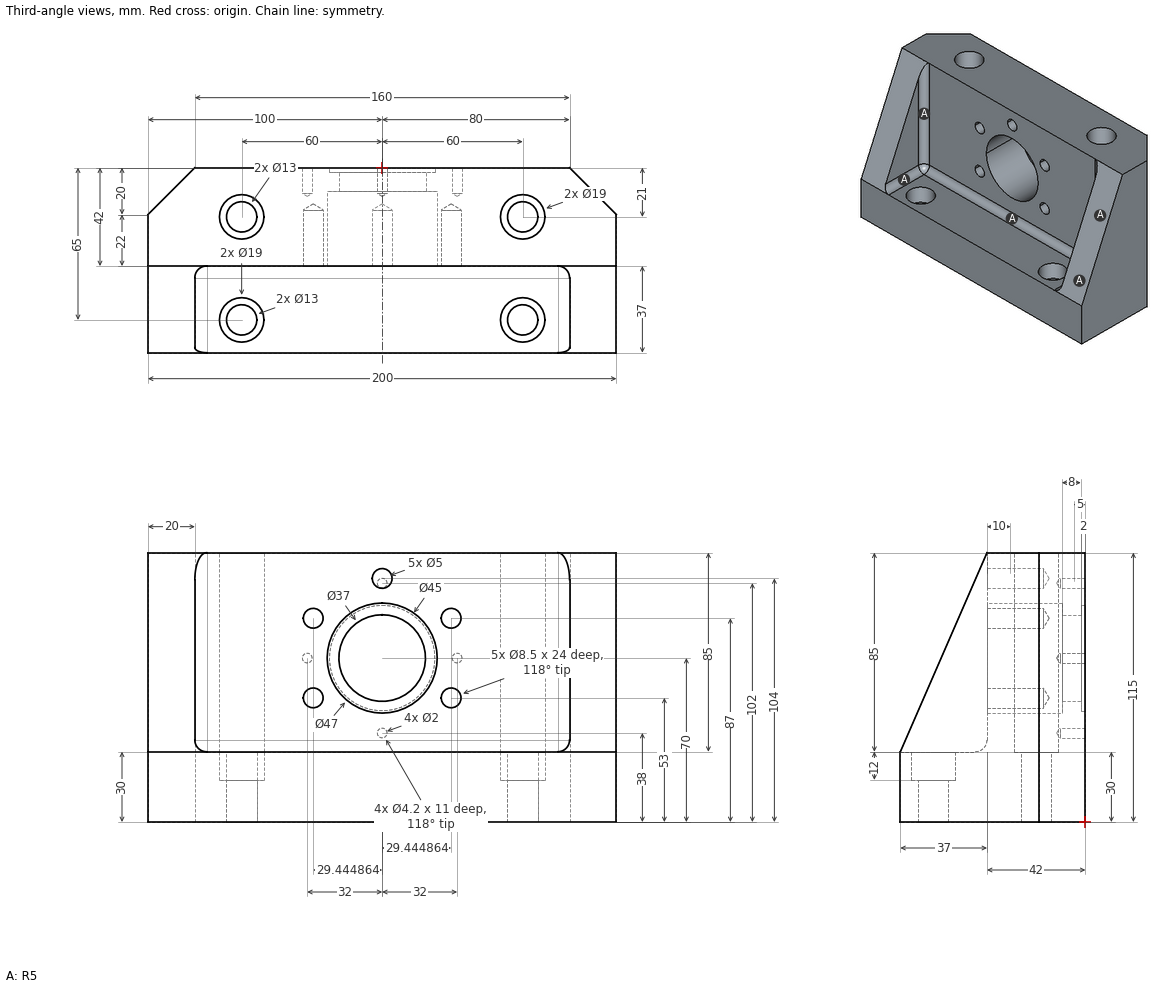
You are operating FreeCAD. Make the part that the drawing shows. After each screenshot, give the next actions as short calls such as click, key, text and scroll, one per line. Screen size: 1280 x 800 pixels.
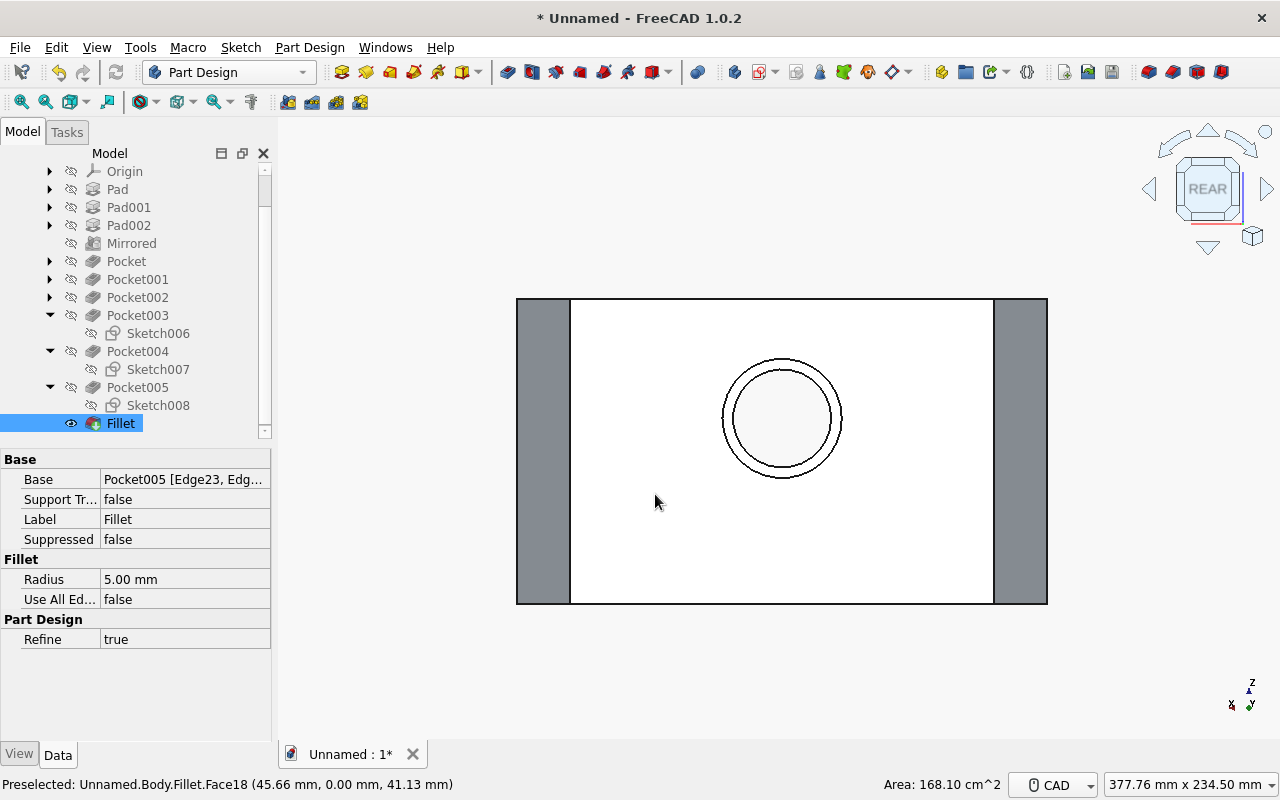
click(760, 72)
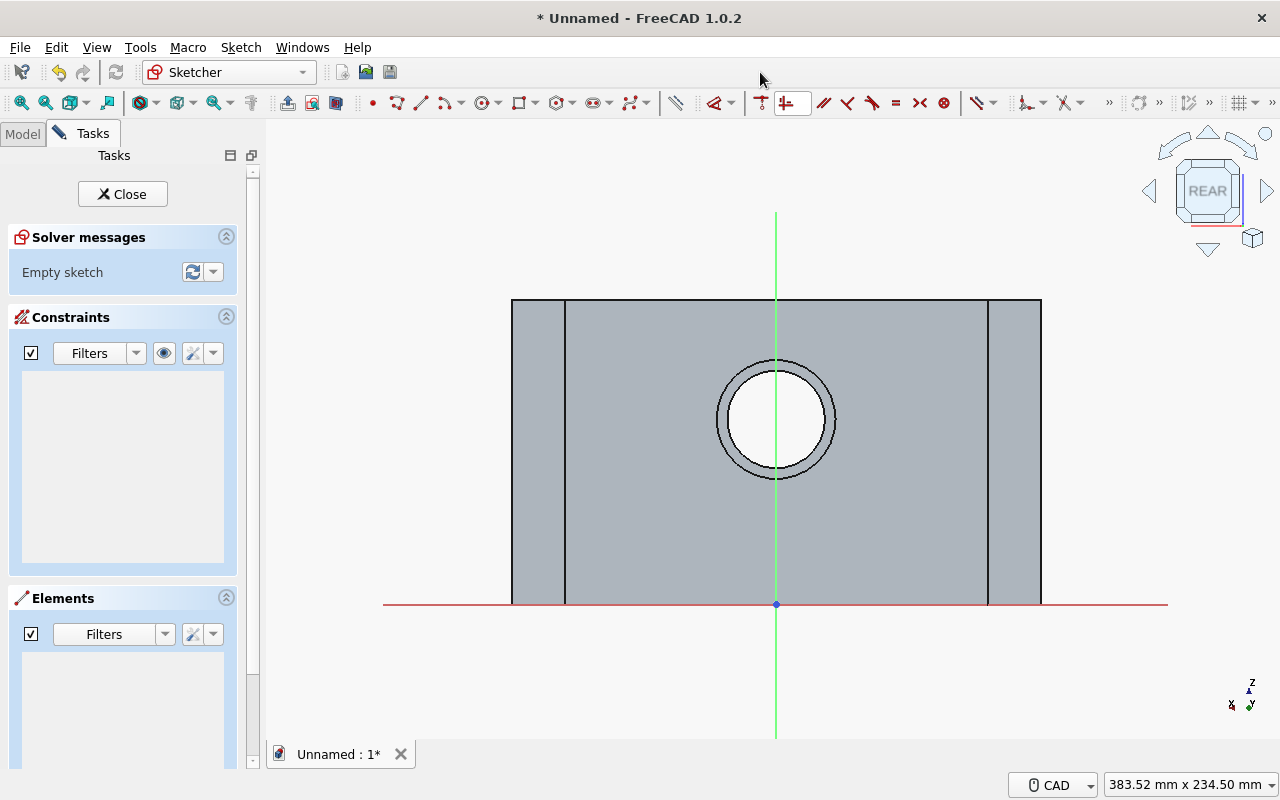
scroll(922, 548, up, 2)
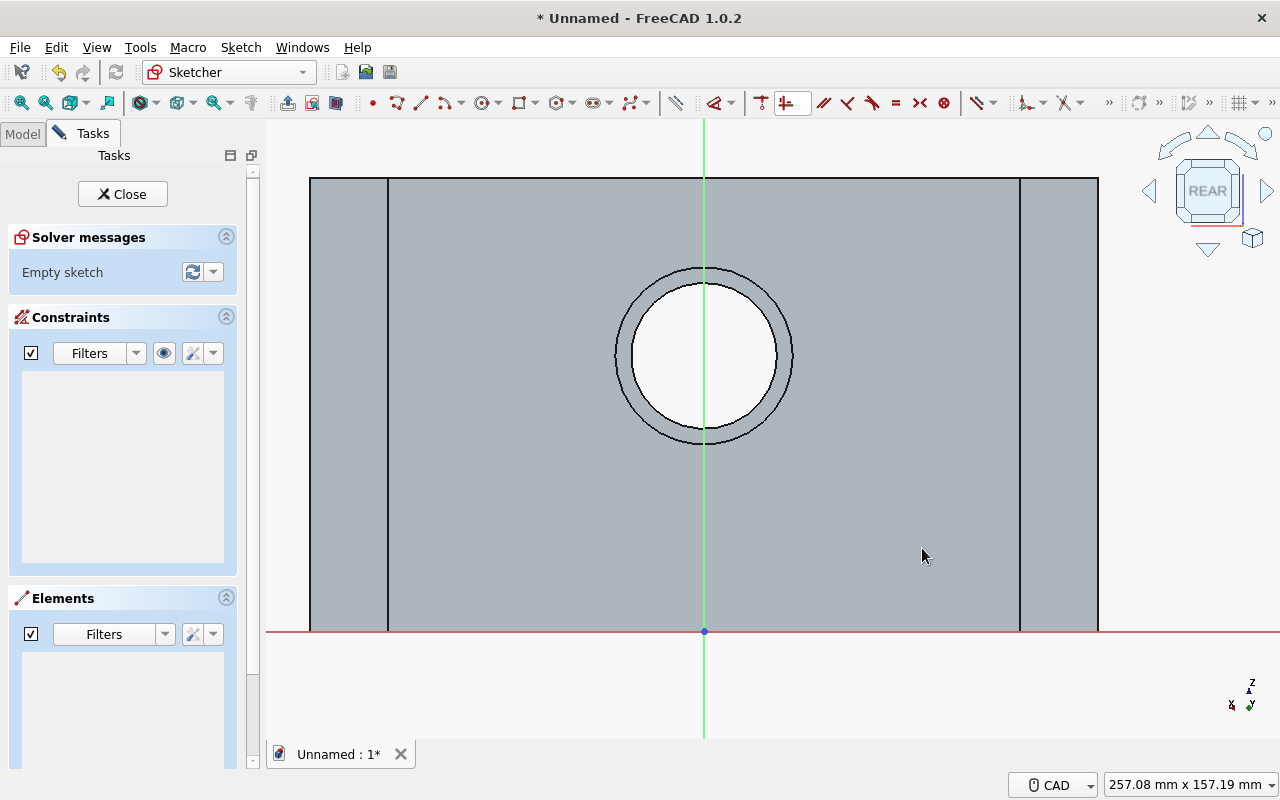
click(482, 104)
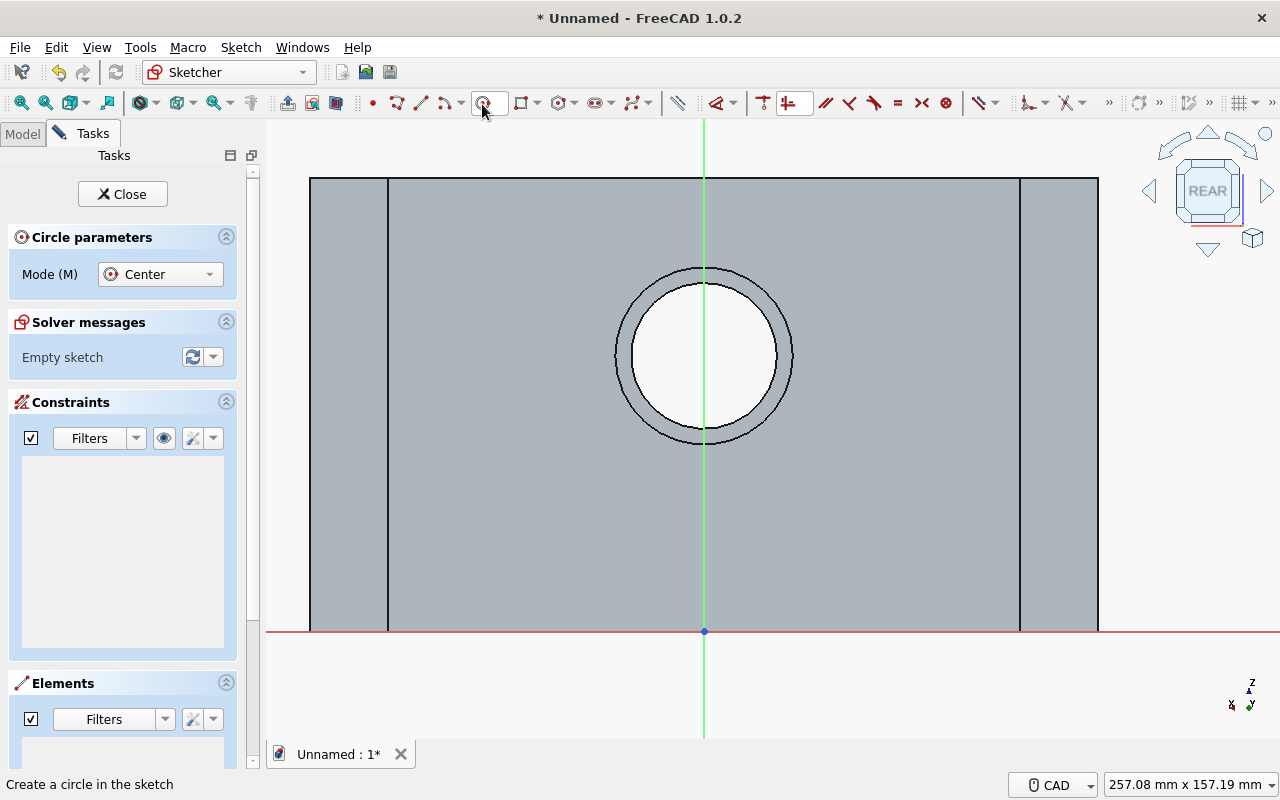
scroll(704, 482, up, 9)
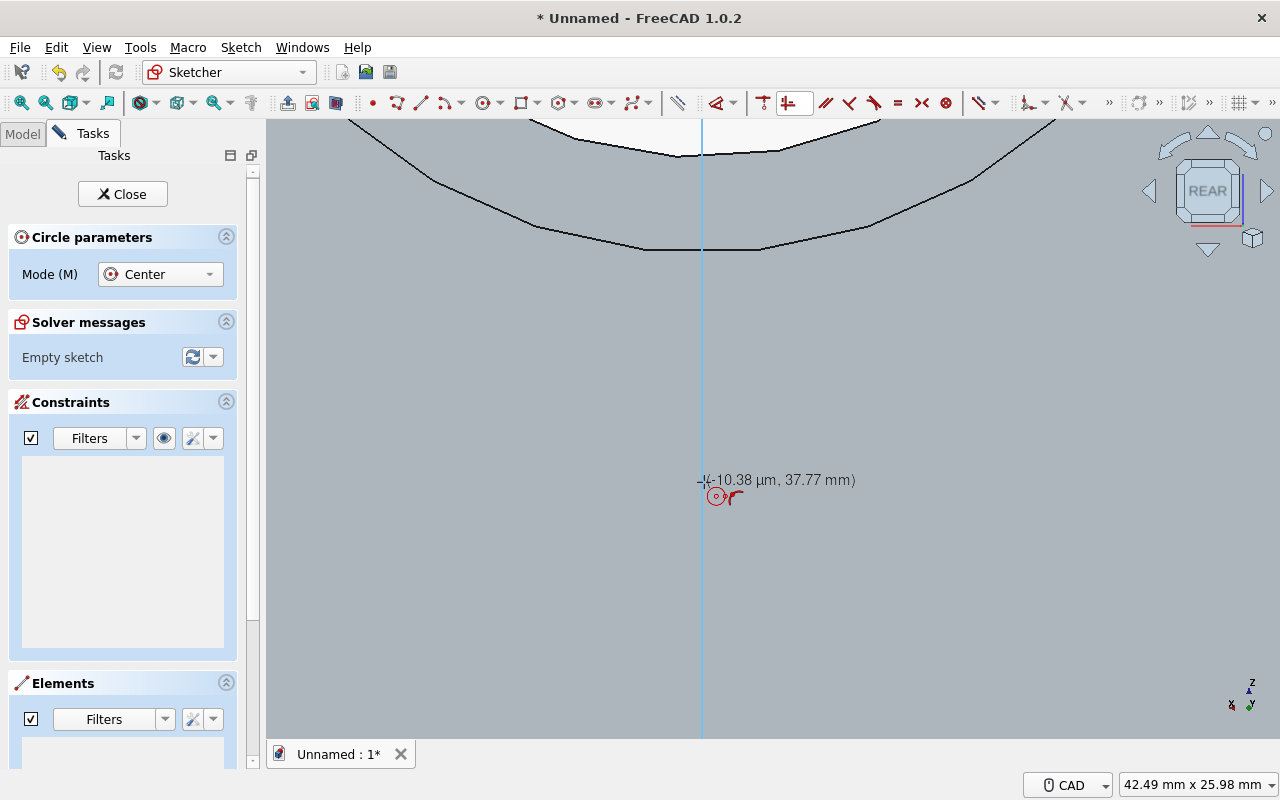
scroll(705, 483, down, 9)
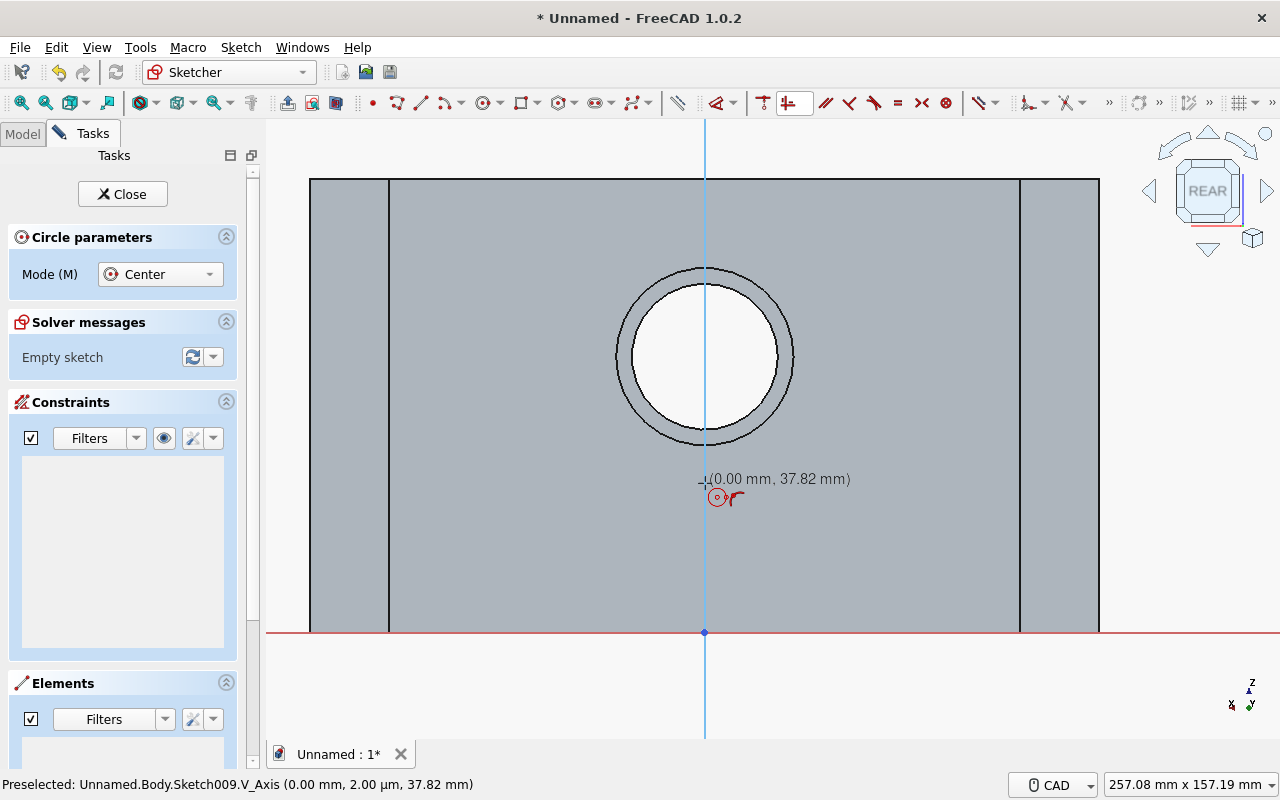
click(705, 483)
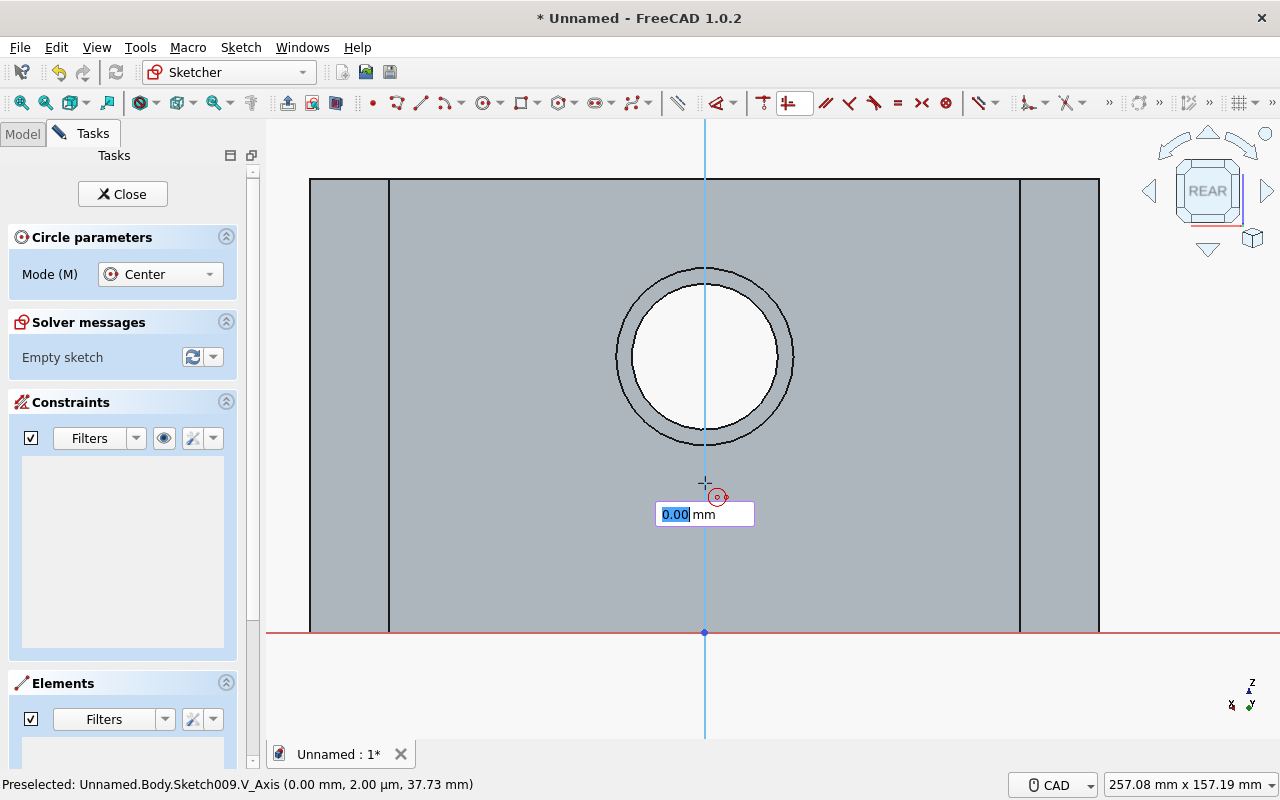
scroll(709, 482, up, 8)
move(705, 478)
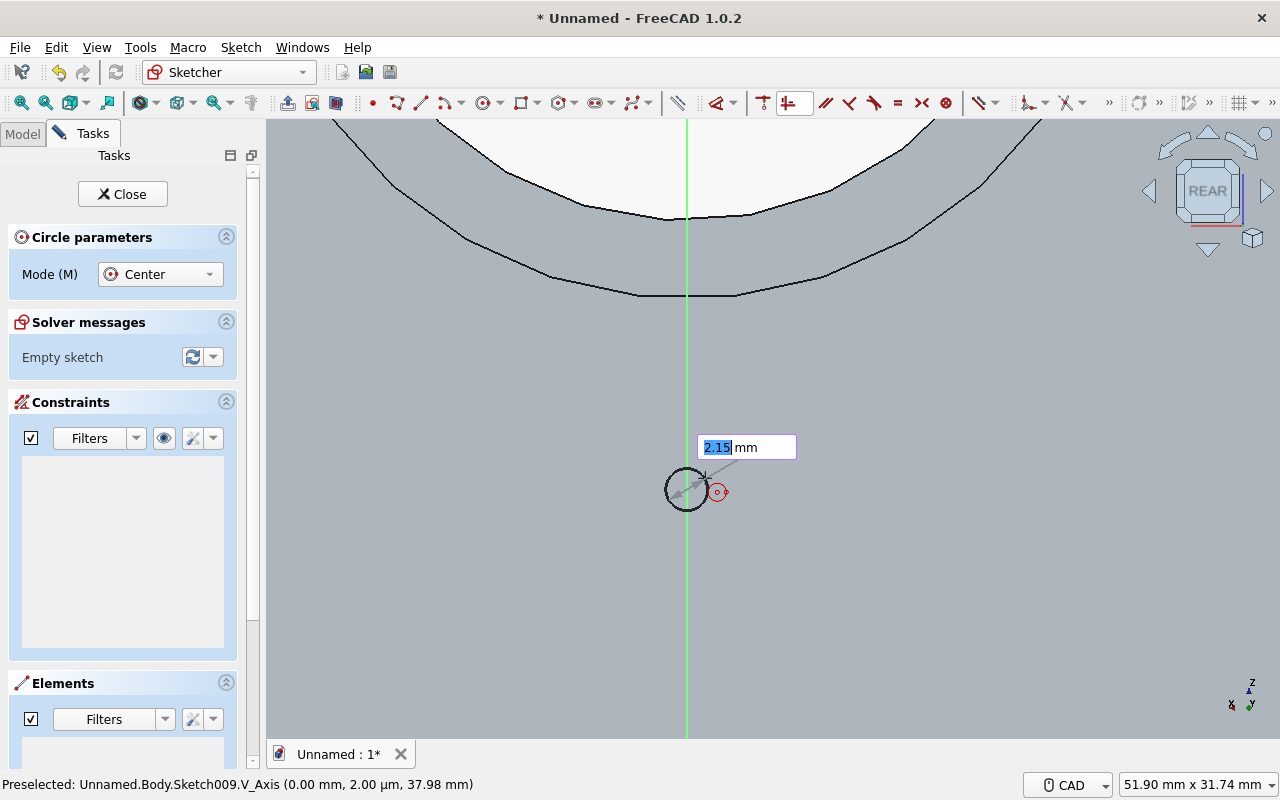
text(2)
key(Return)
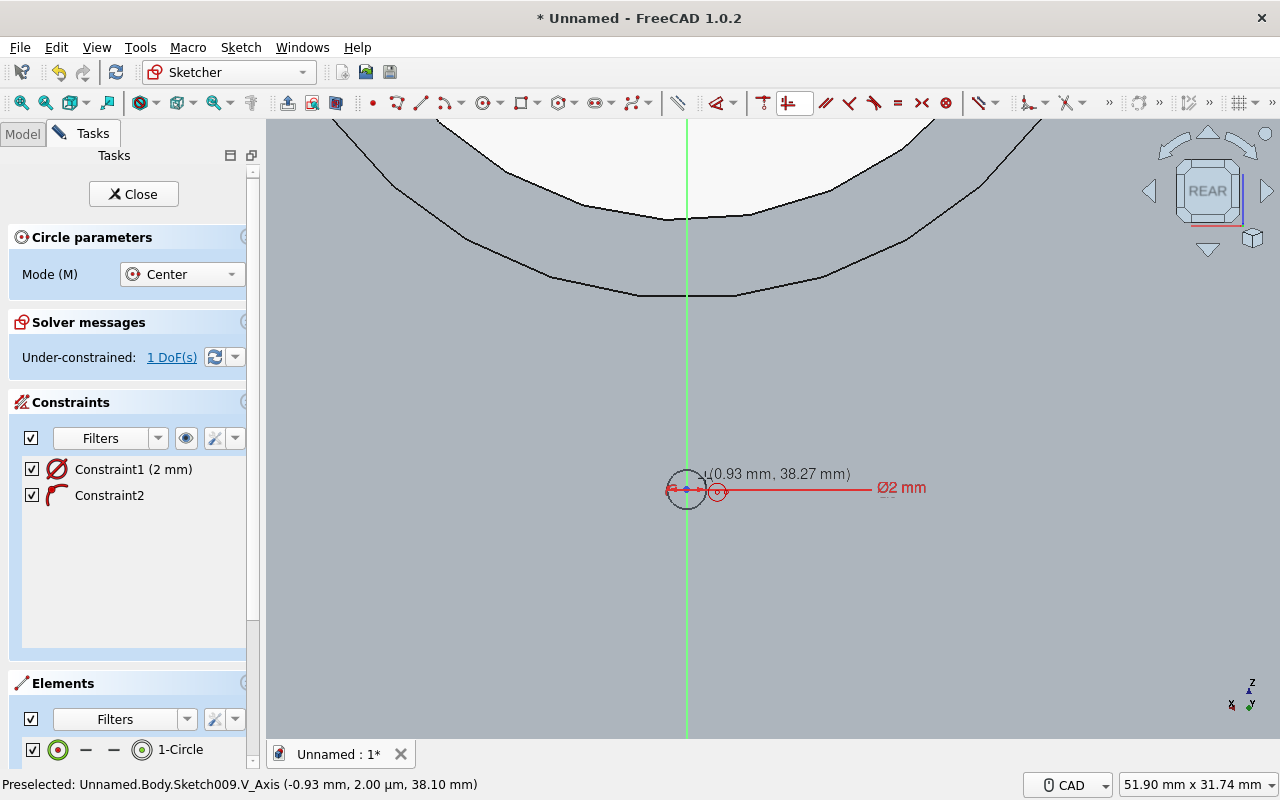
scroll(709, 482, down, 8)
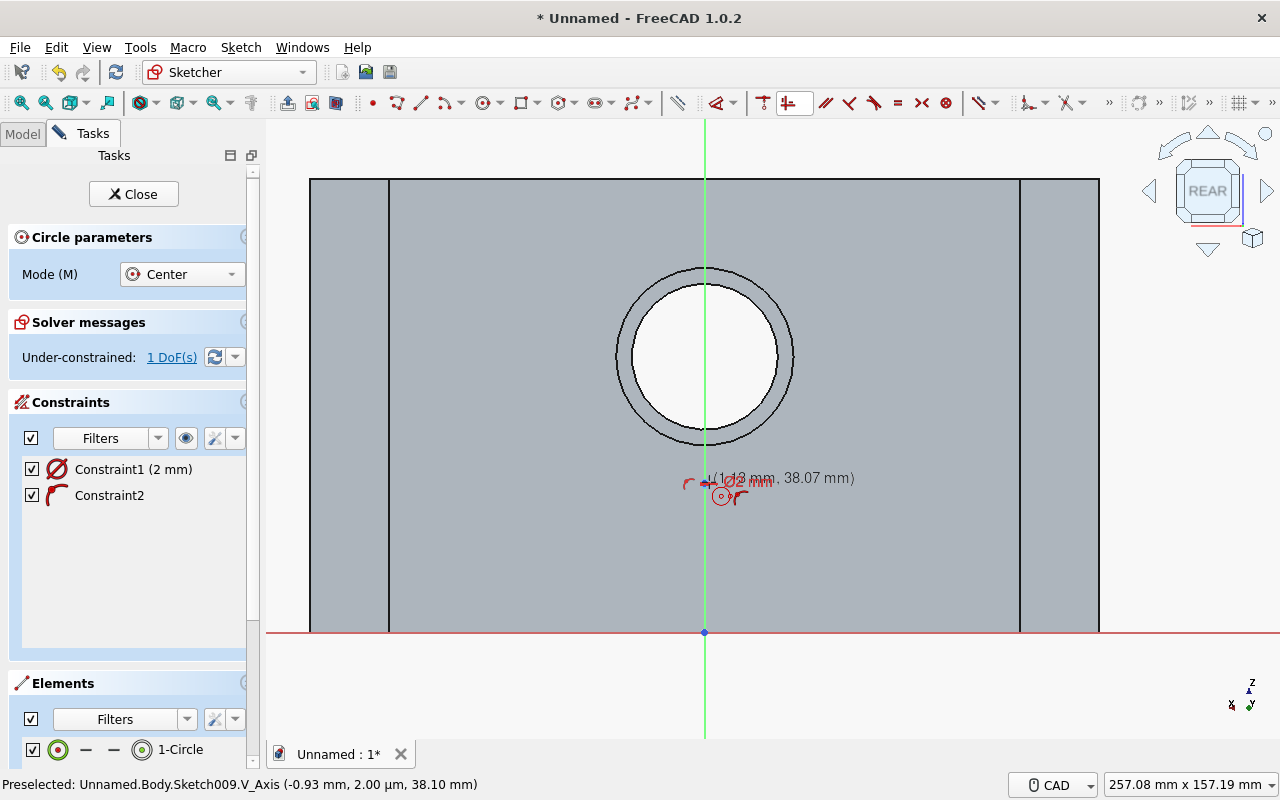
scroll(579, 357, up, 9)